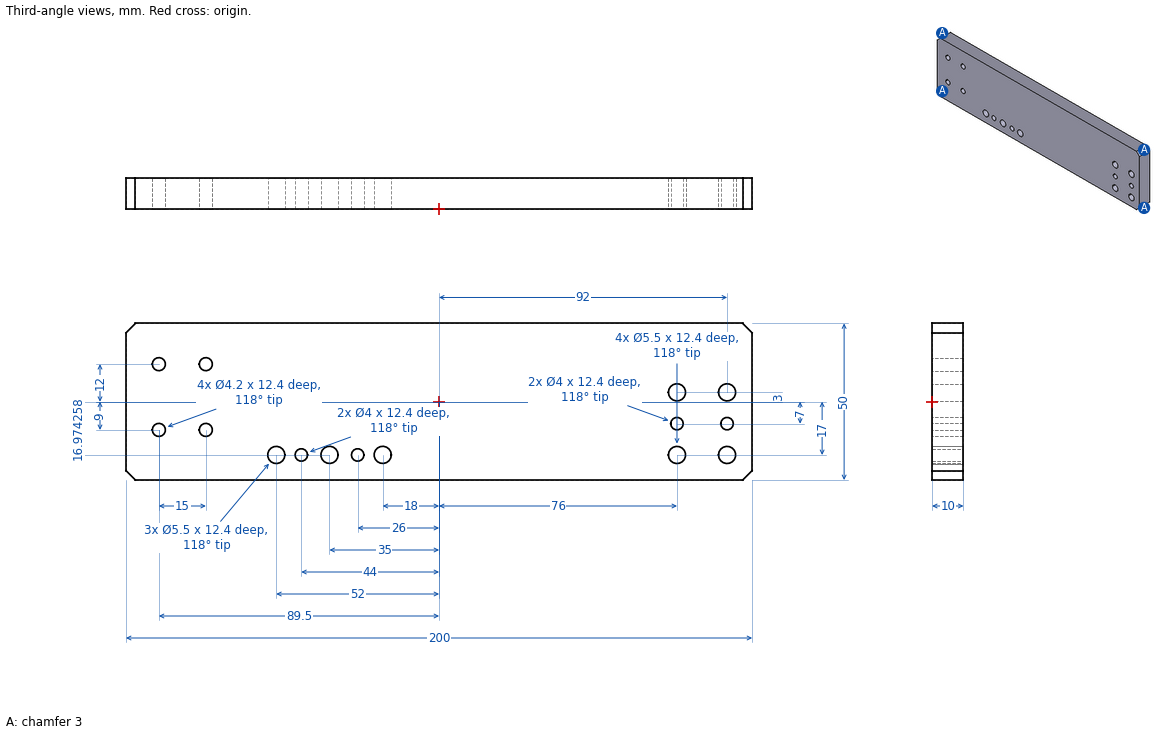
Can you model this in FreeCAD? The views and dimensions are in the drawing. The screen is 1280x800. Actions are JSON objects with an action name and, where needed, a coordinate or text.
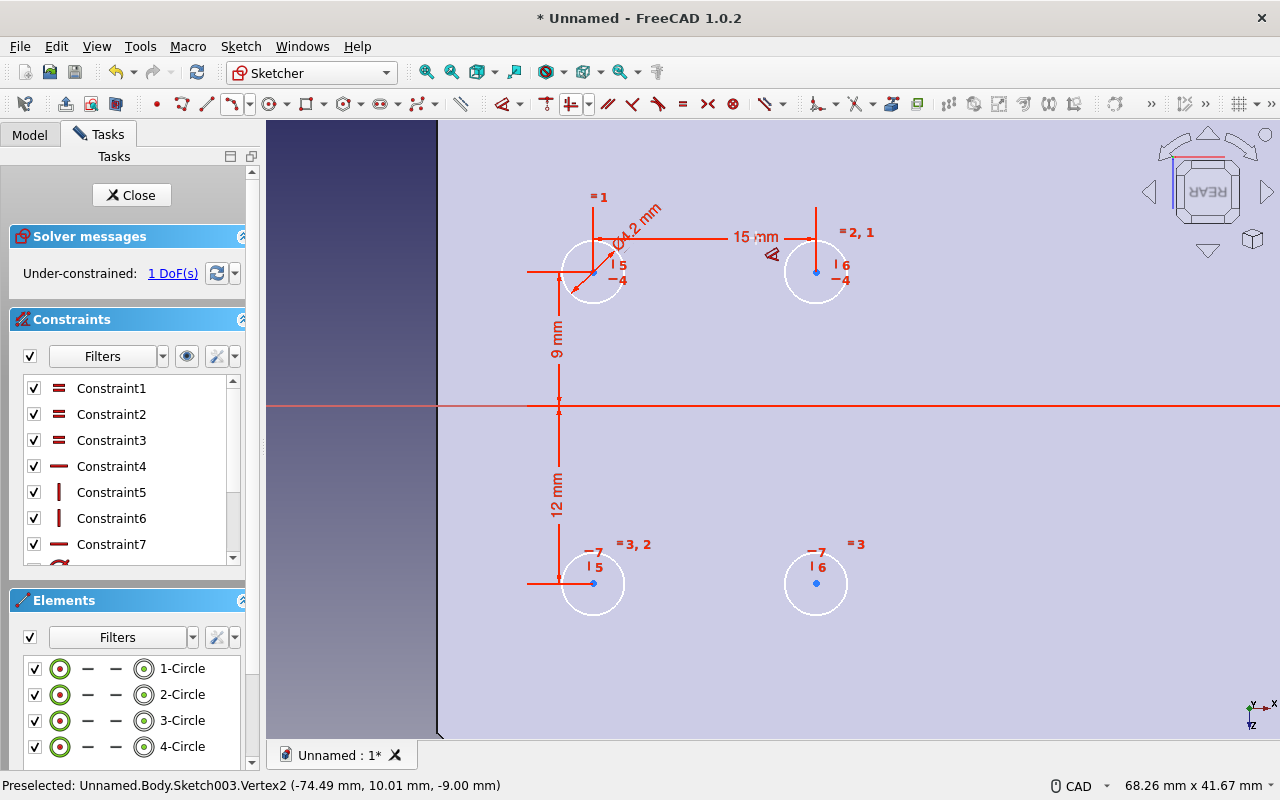
{"action": "left_click", "coordinate": [593, 272]}
{"action": "left_click", "coordinate": [854, 238]}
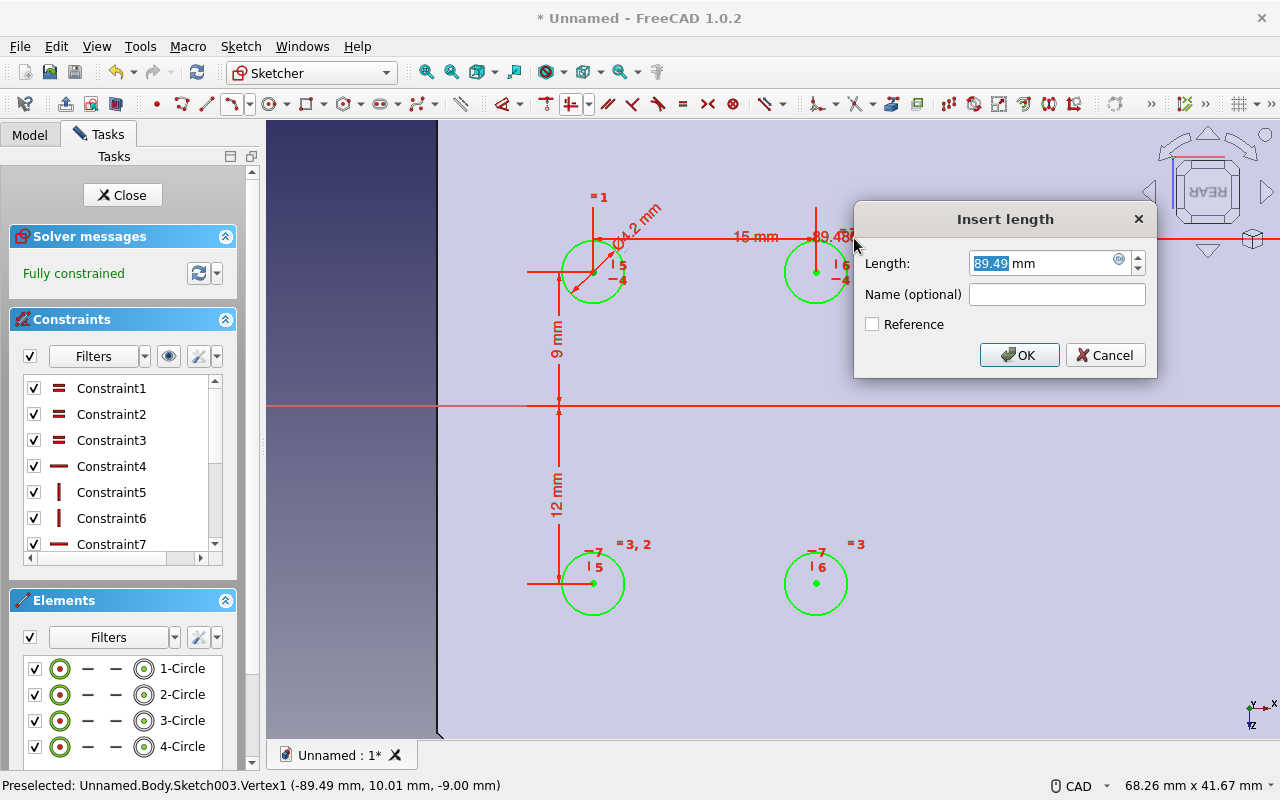
{"action": "type", "text": "89.5"}
{"action": "key", "text": "Return"}
{"action": "key", "text": "Escape"}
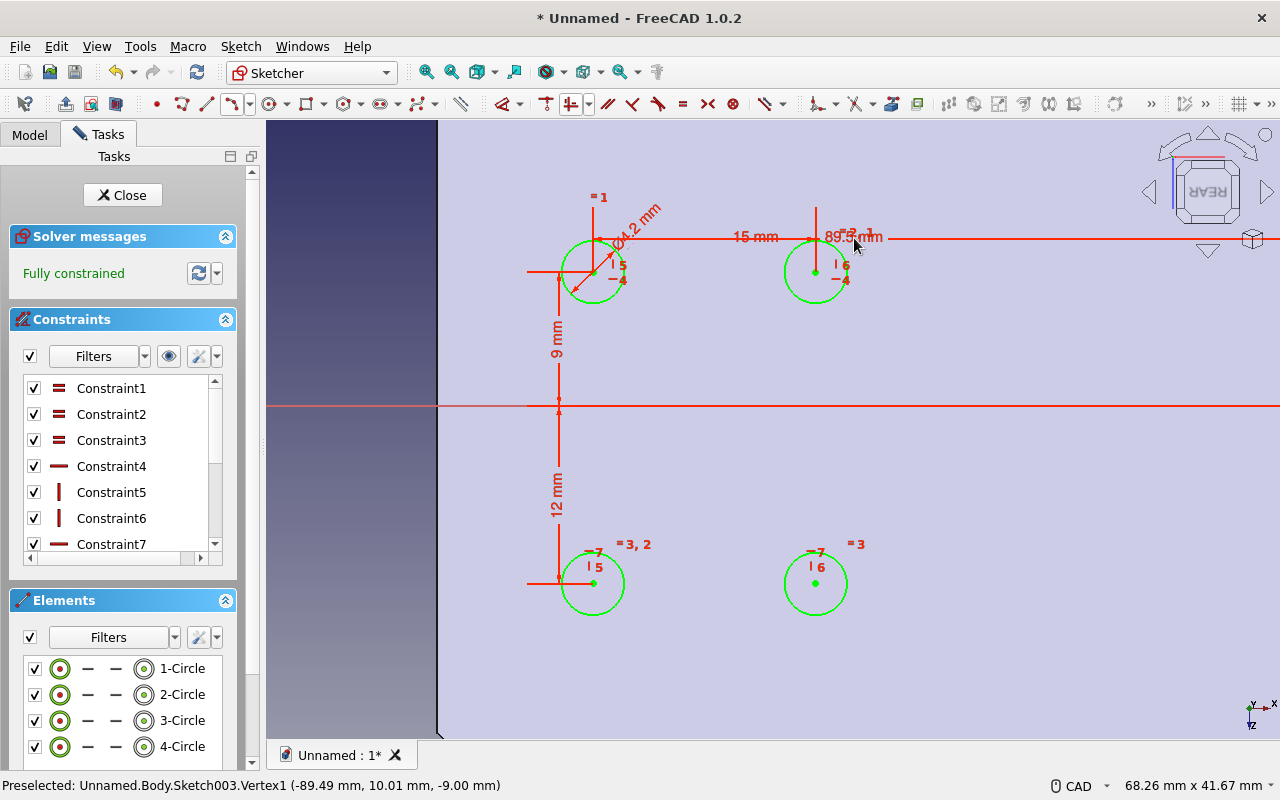
{"action": "left_click", "coordinate": [123, 195]}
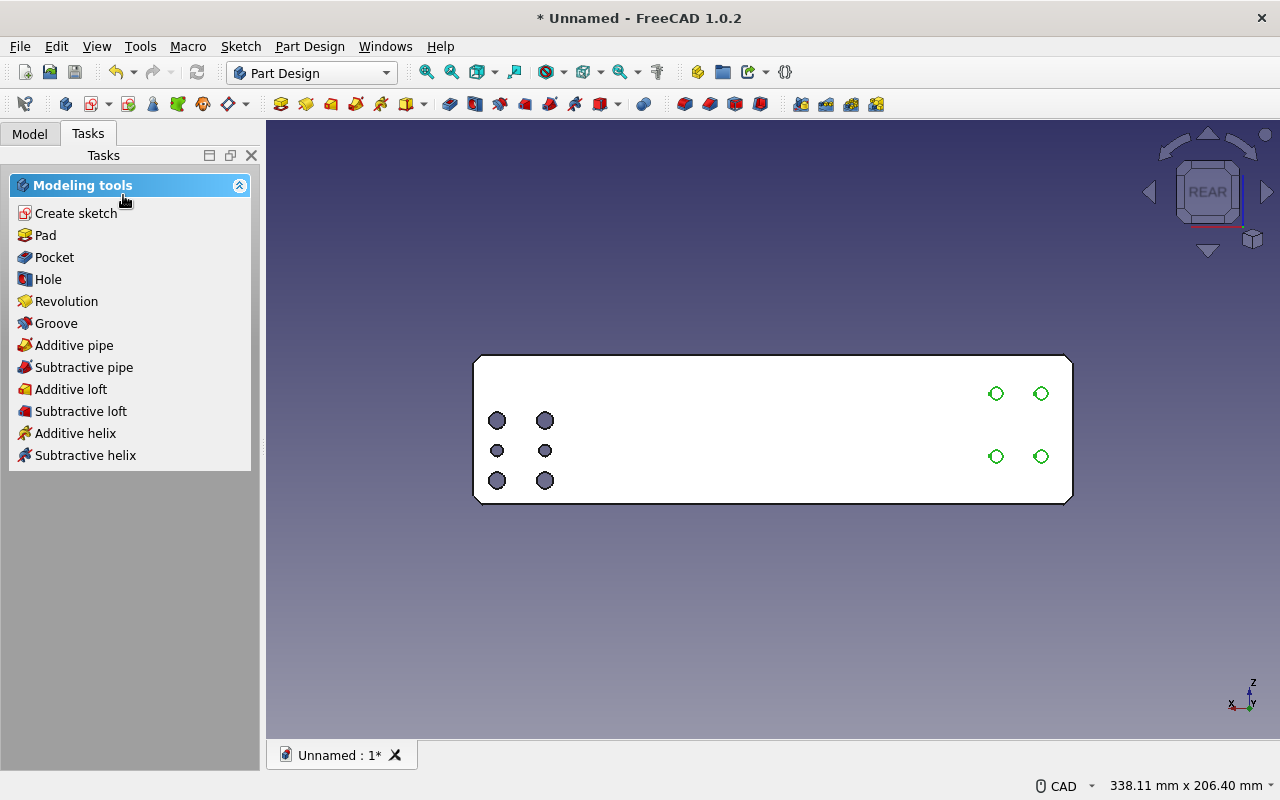
{"action": "left_click", "coordinate": [475, 104]}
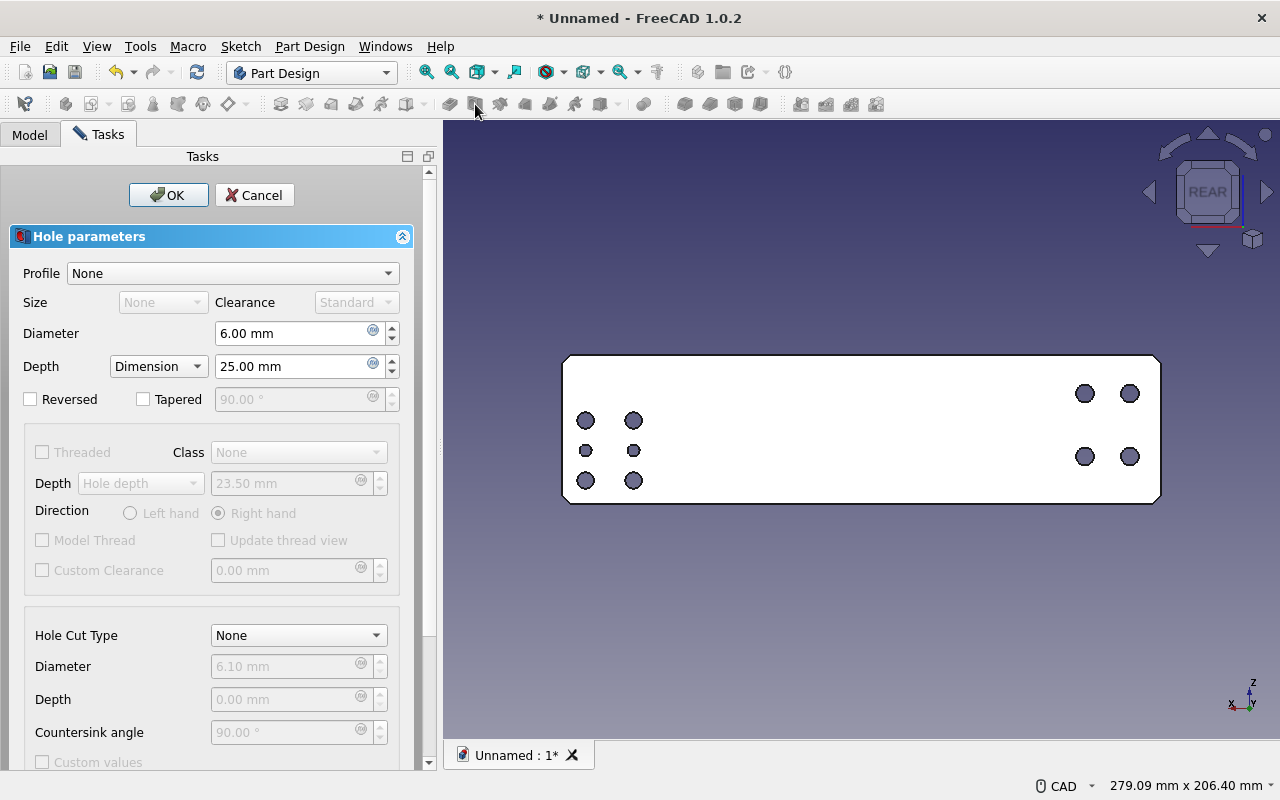
{"action": "triple_click", "coordinate": [300, 334]}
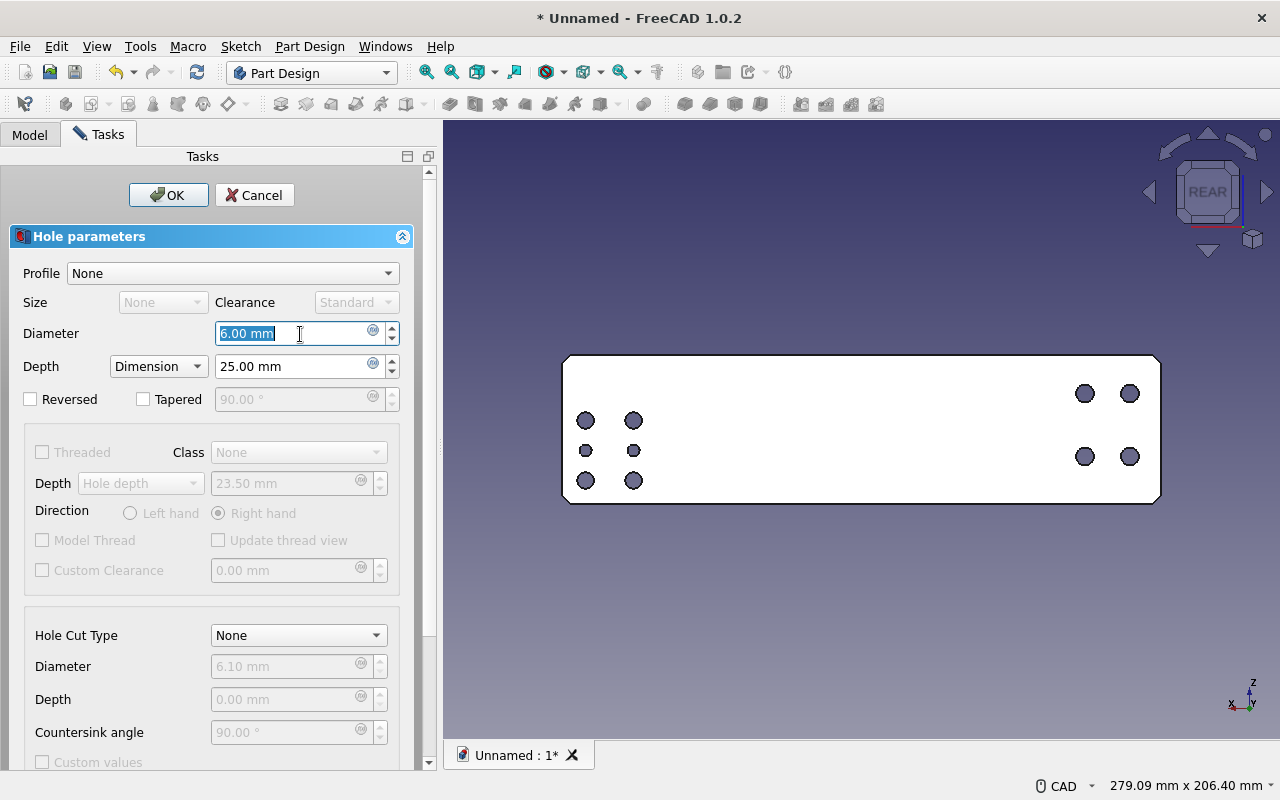
{"action": "type", "text": "4.2"}
{"action": "key", "text": "Tab"}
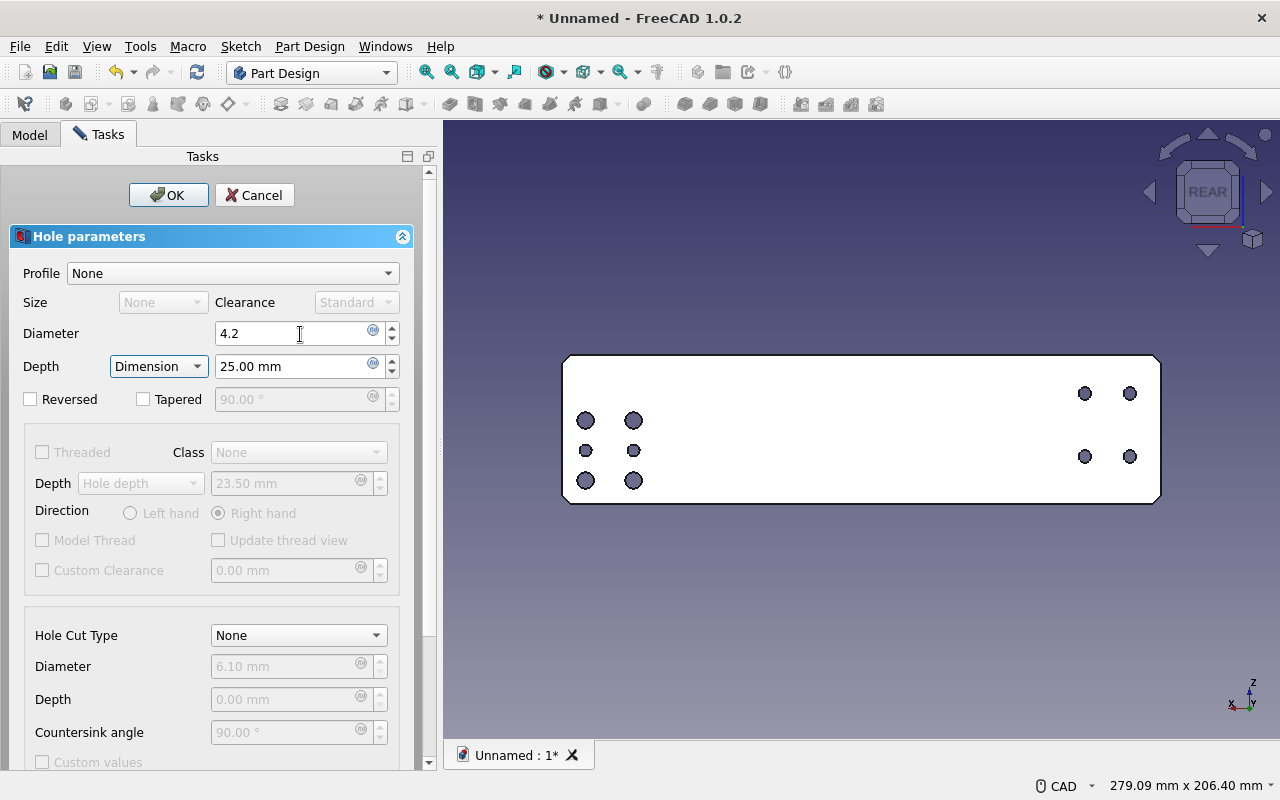
{"action": "triple_click", "coordinate": [300, 366]}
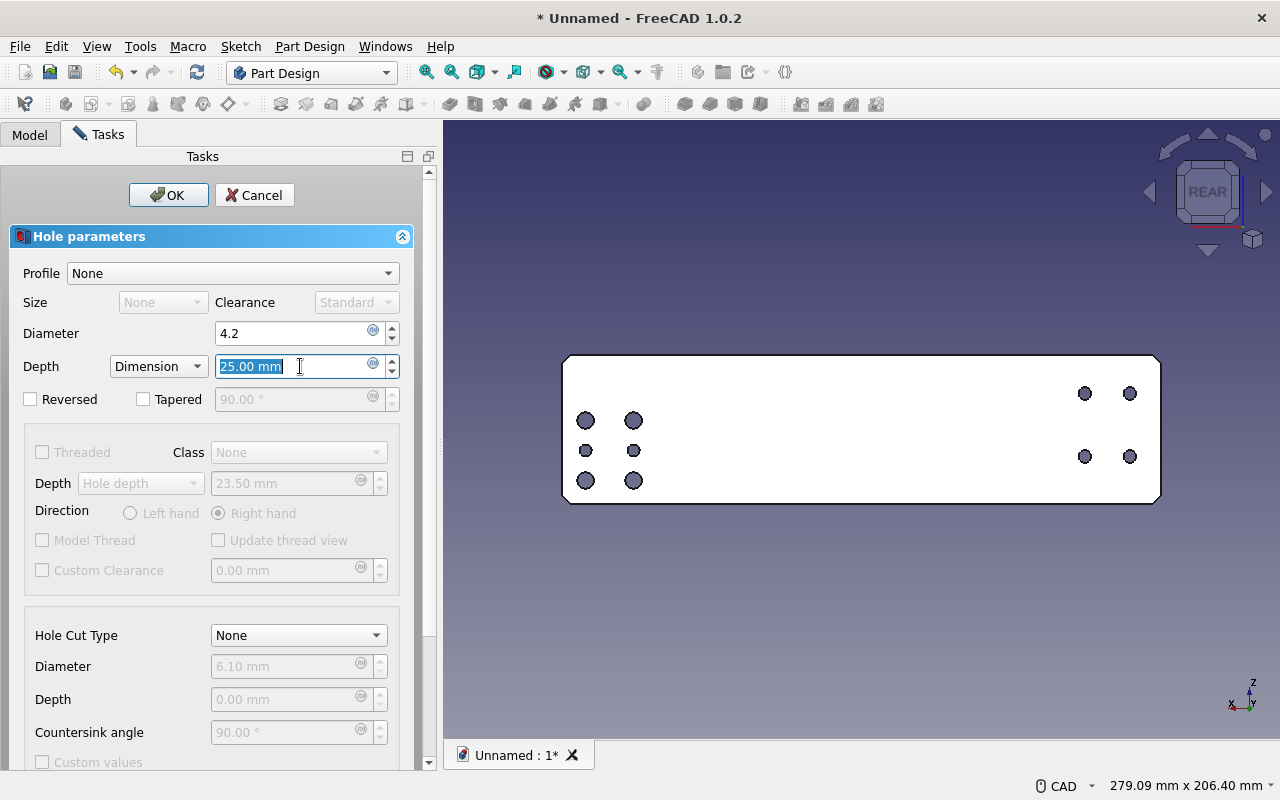
{"action": "type", "text": "12.4"}
{"action": "key", "text": "Tab"}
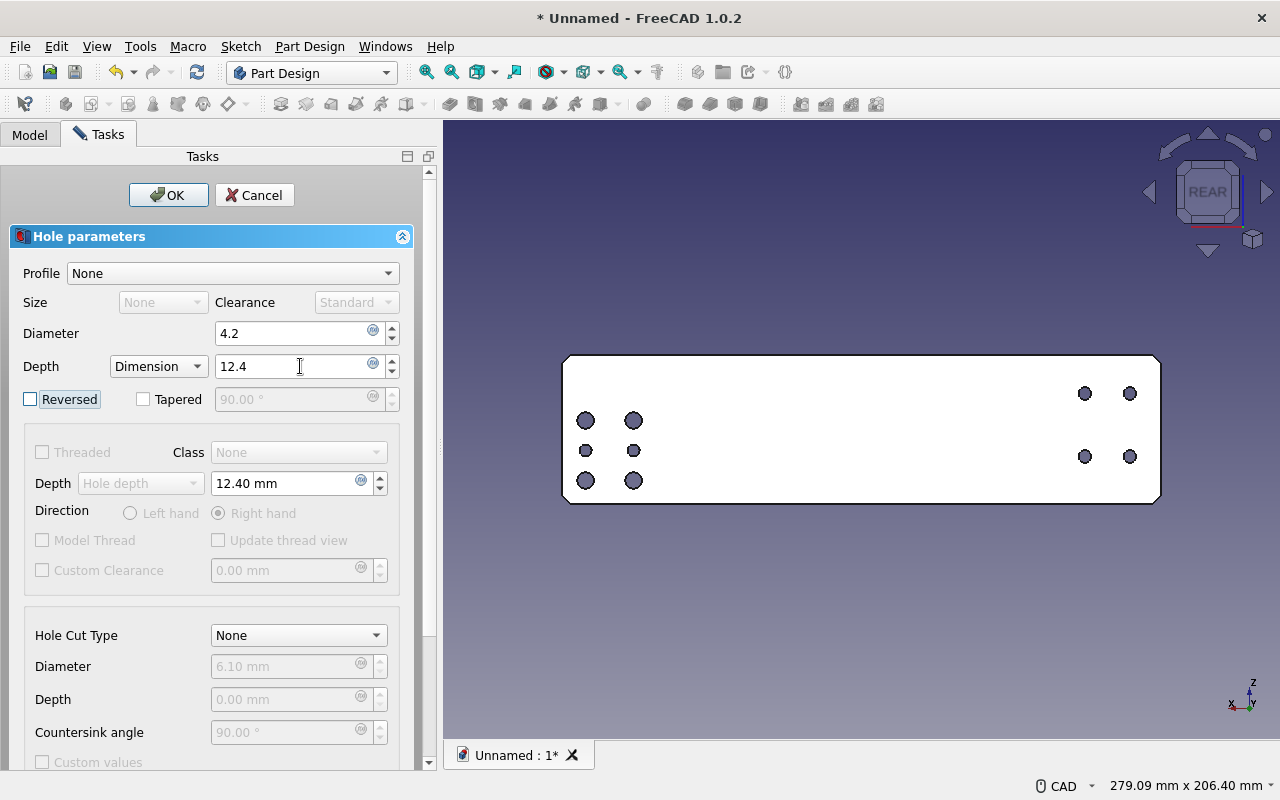
{"action": "left_click", "coordinate": [169, 195]}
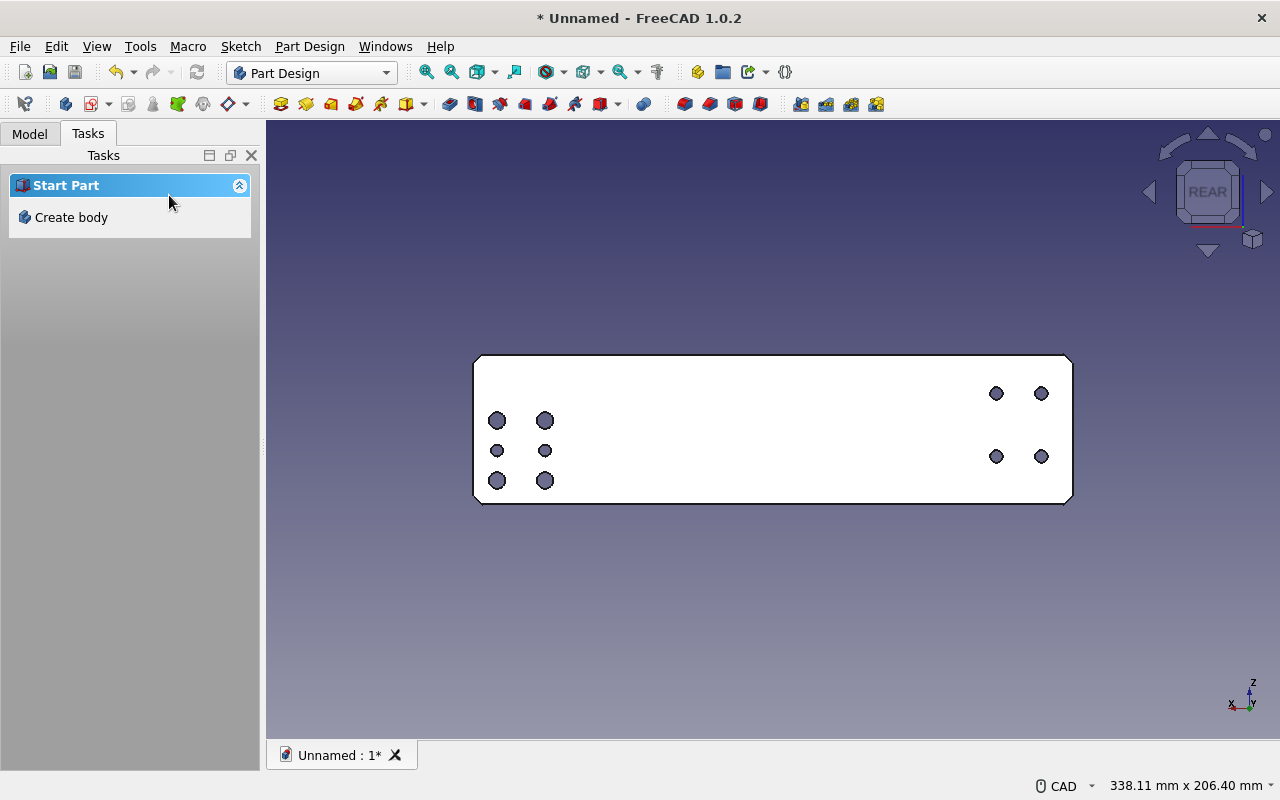
{"action": "left_click", "coordinate": [90, 104]}